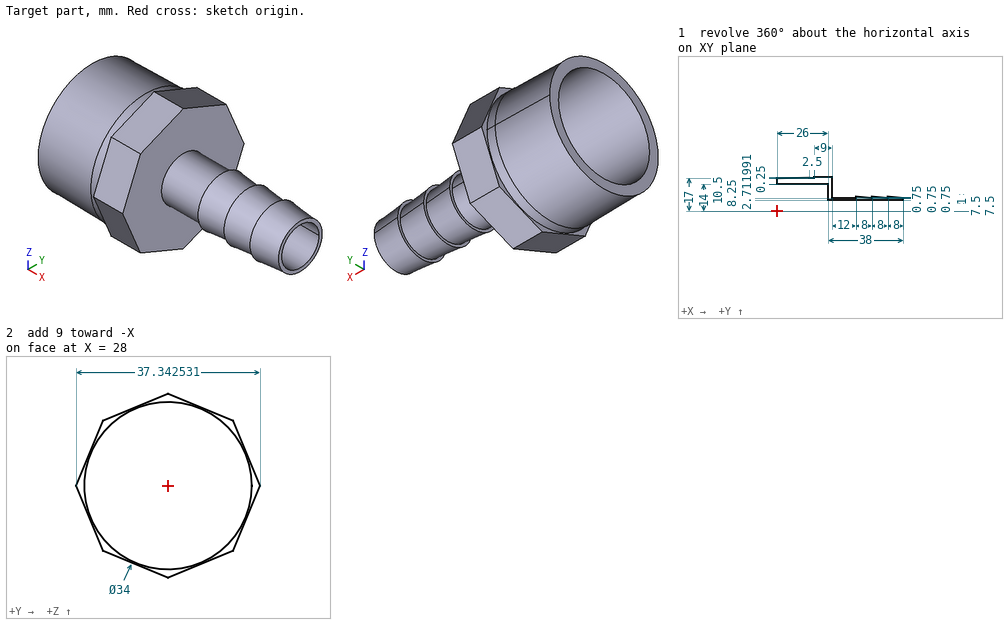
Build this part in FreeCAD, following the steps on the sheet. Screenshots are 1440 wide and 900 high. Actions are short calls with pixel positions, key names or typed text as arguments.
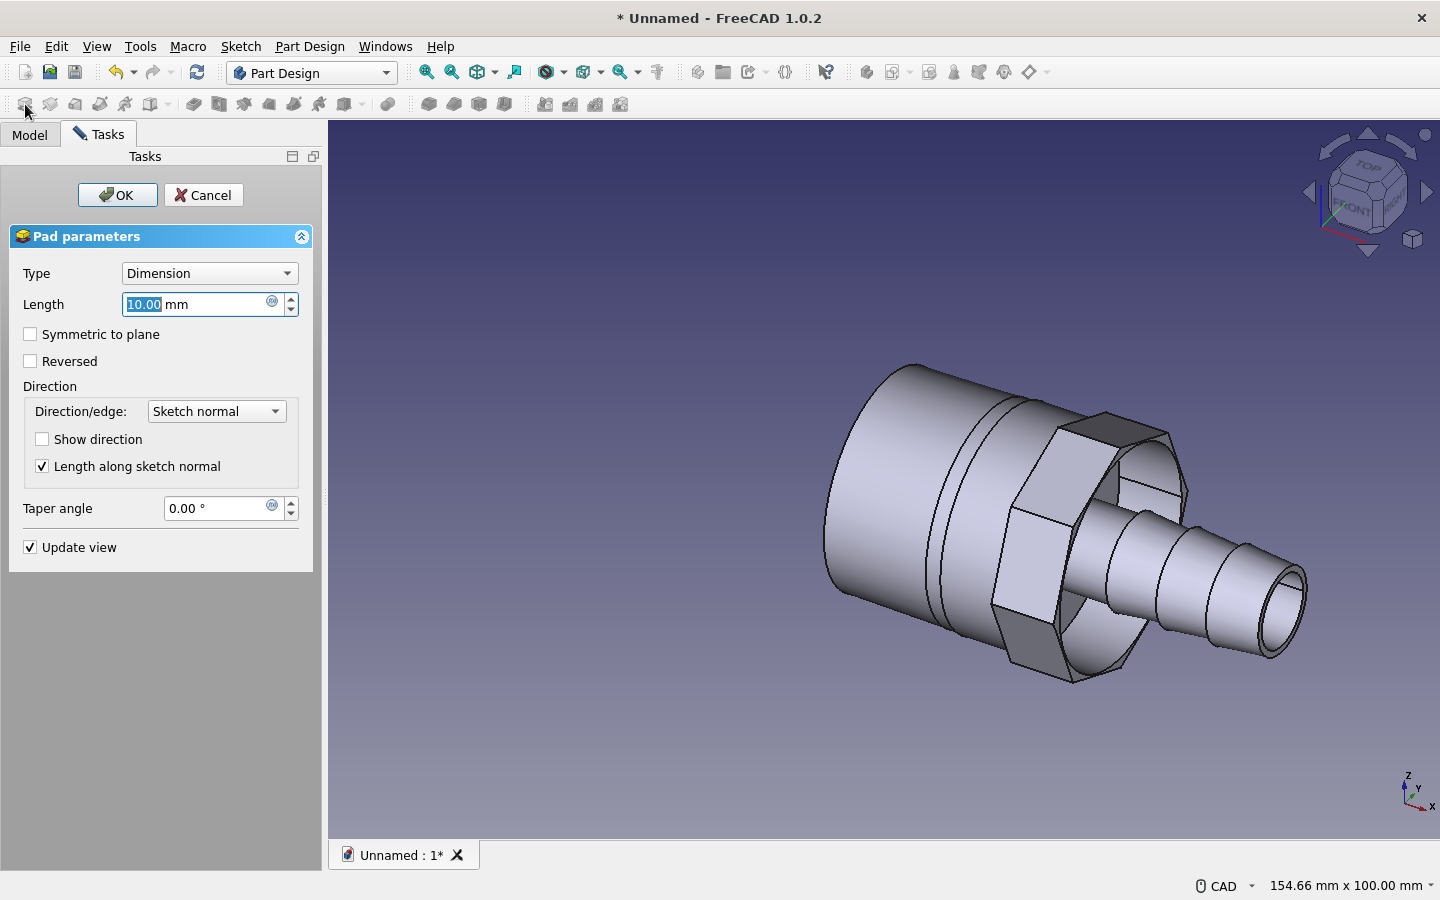
text(9)
key(Tab)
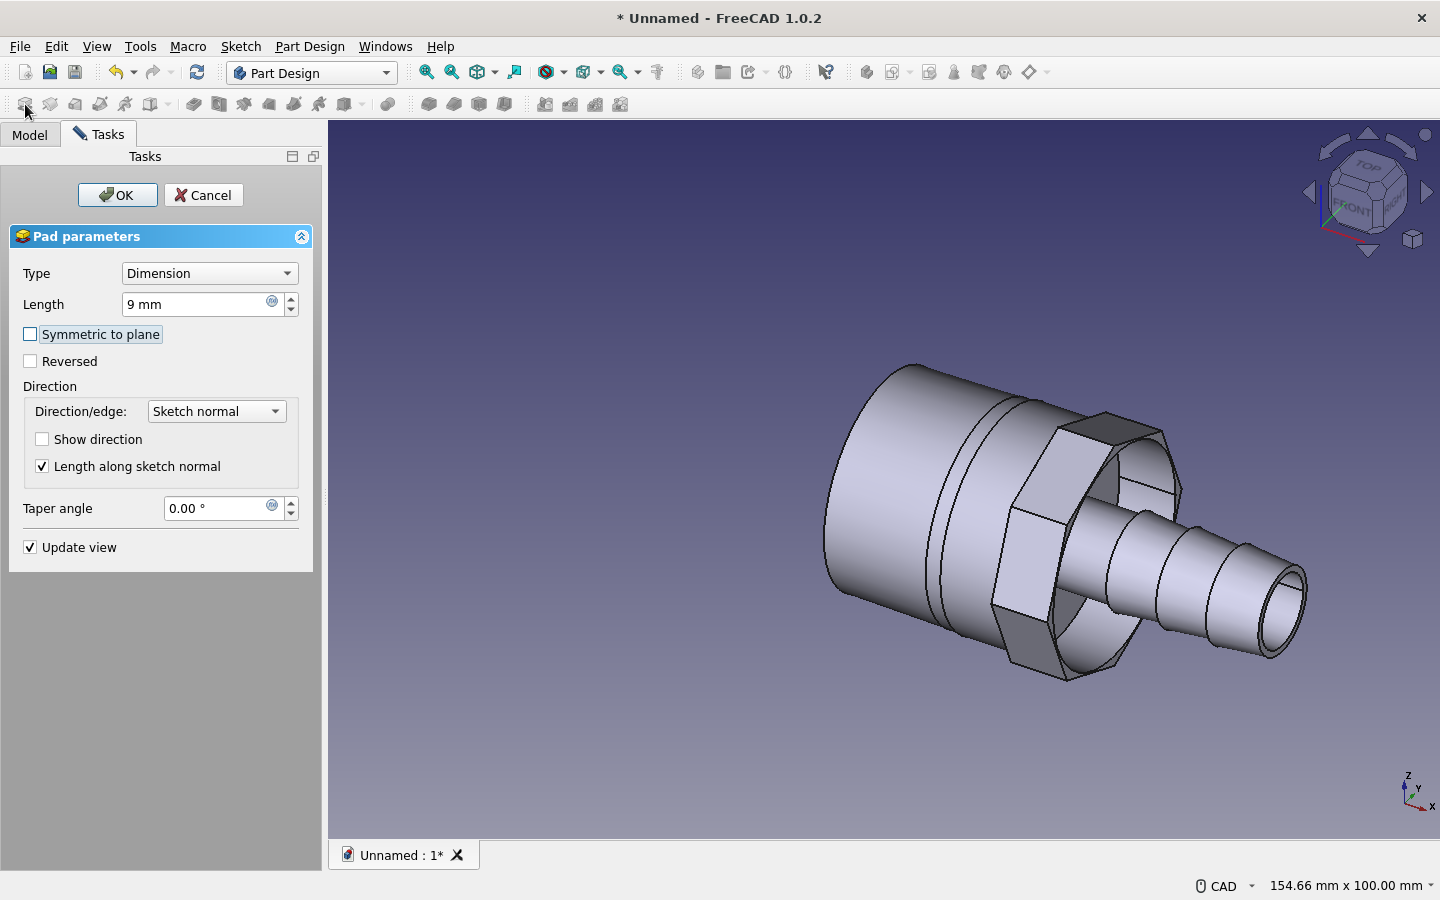
click(31, 361)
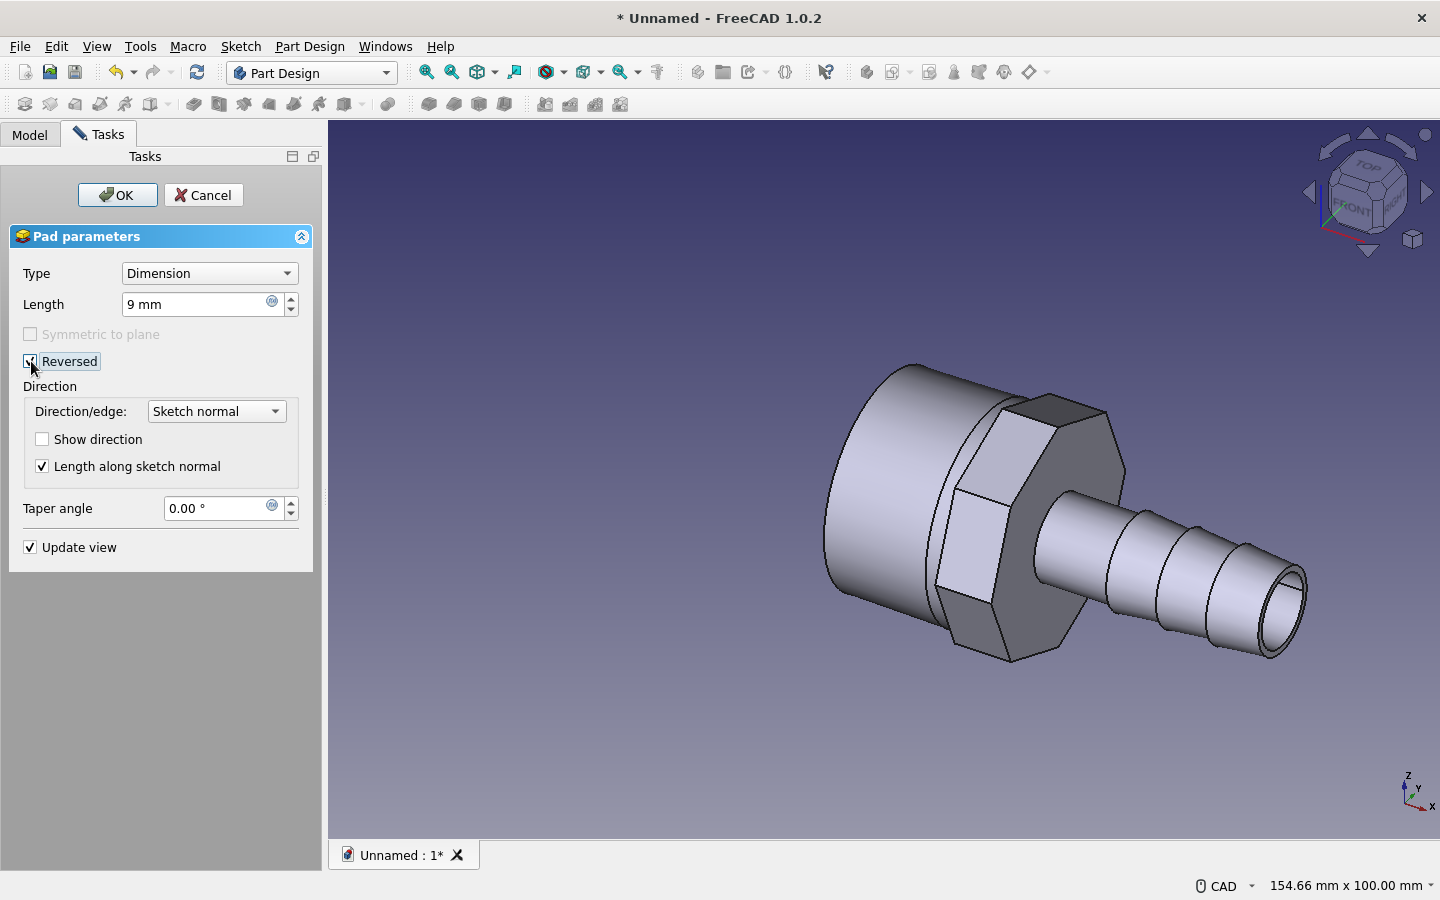
click(118, 195)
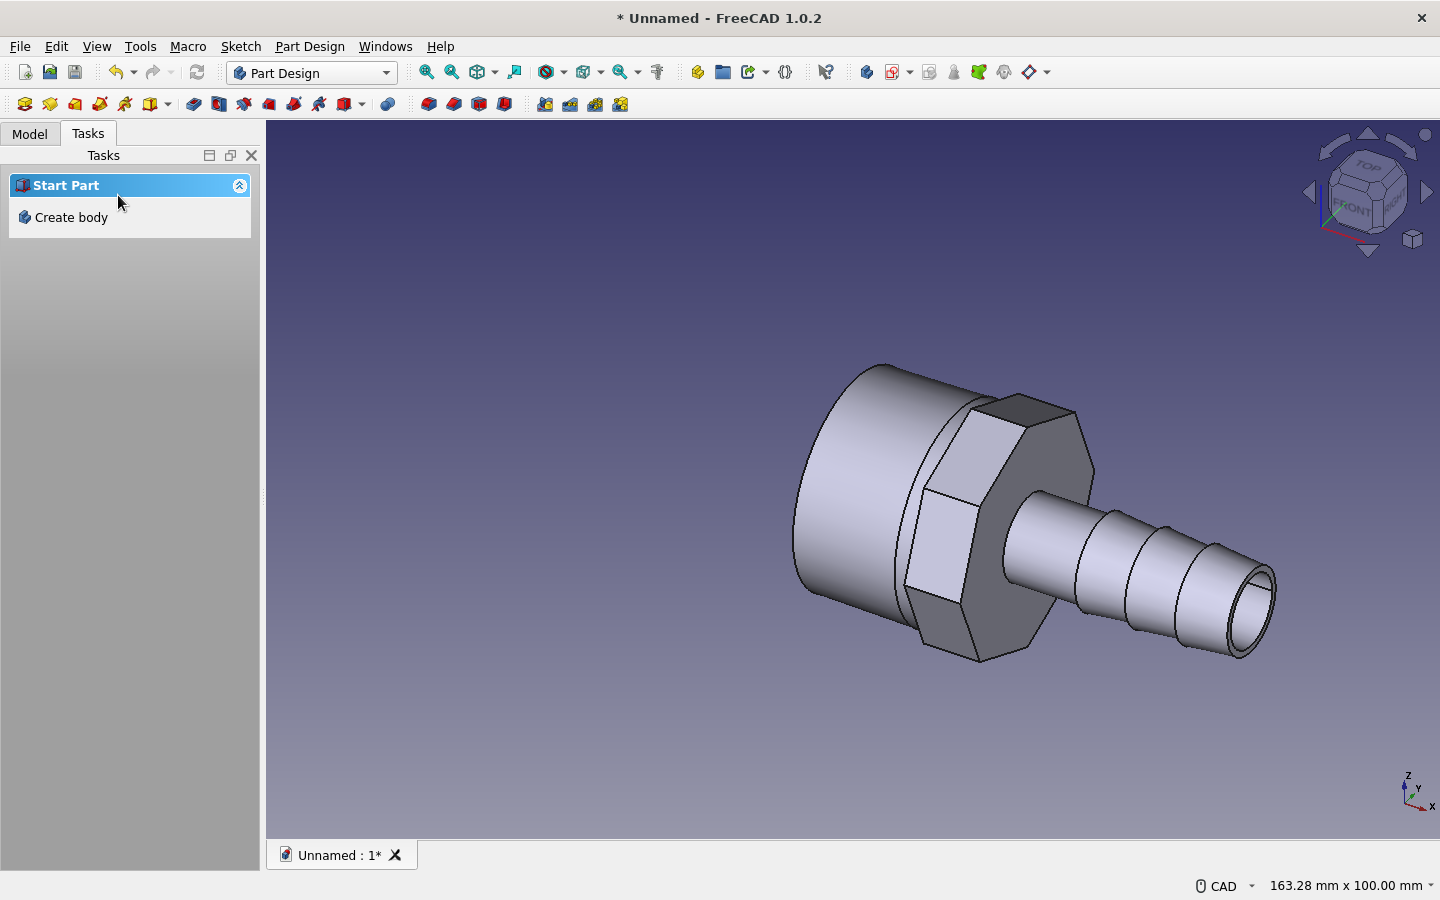
key(0)